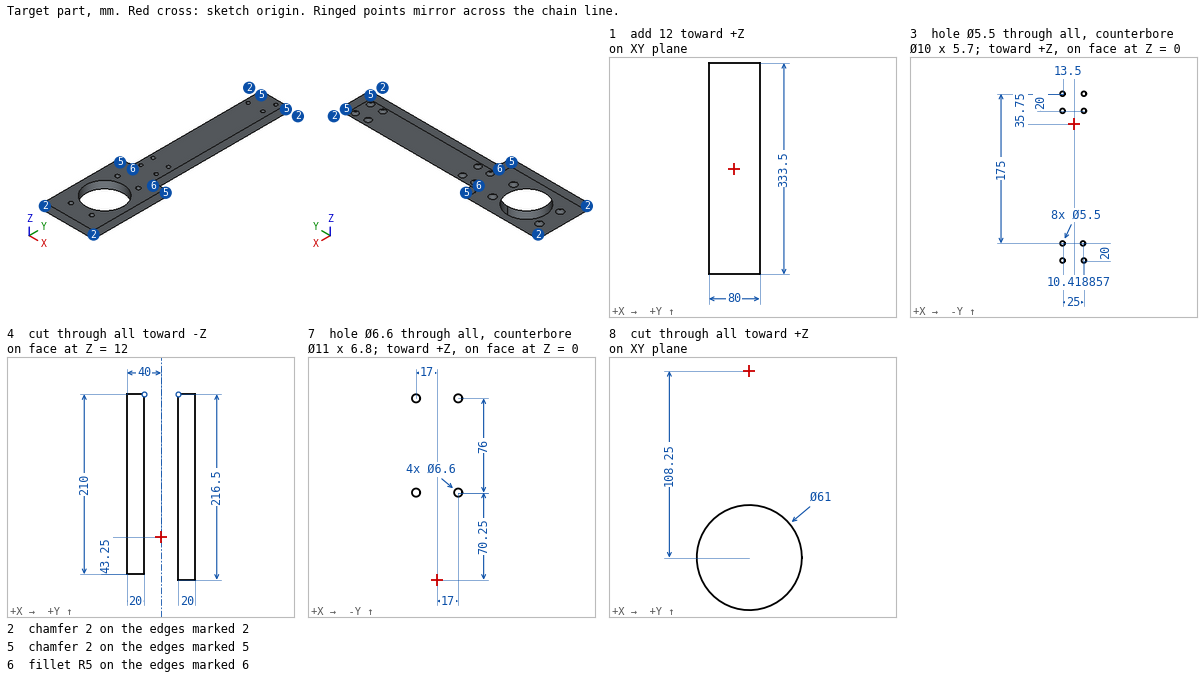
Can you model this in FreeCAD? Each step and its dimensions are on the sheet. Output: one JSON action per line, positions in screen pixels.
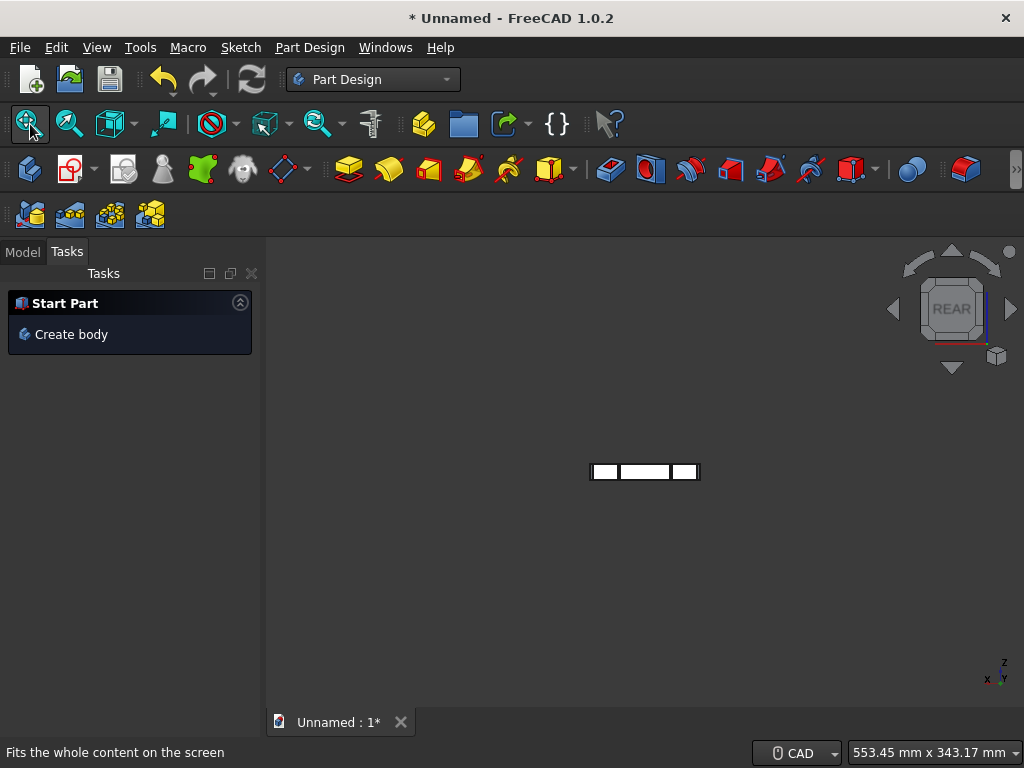
{"action": "scroll", "coordinate": [672, 471], "scroll_direction": "up", "scroll_amount": 5}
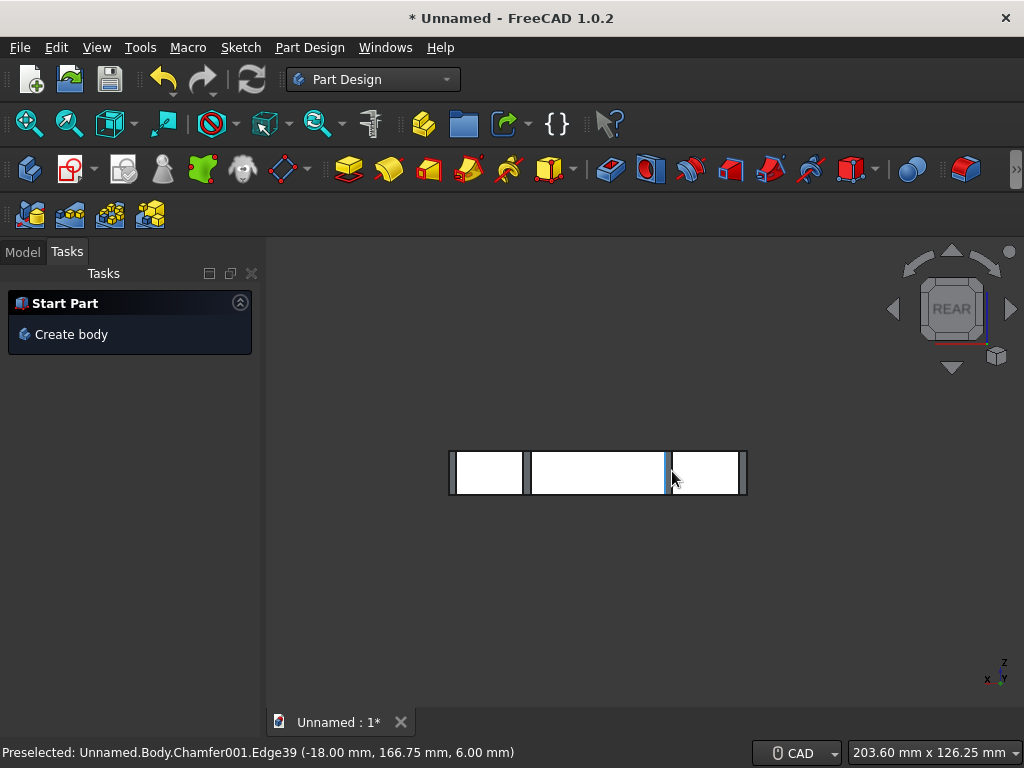
{"action": "key", "text": "v f"}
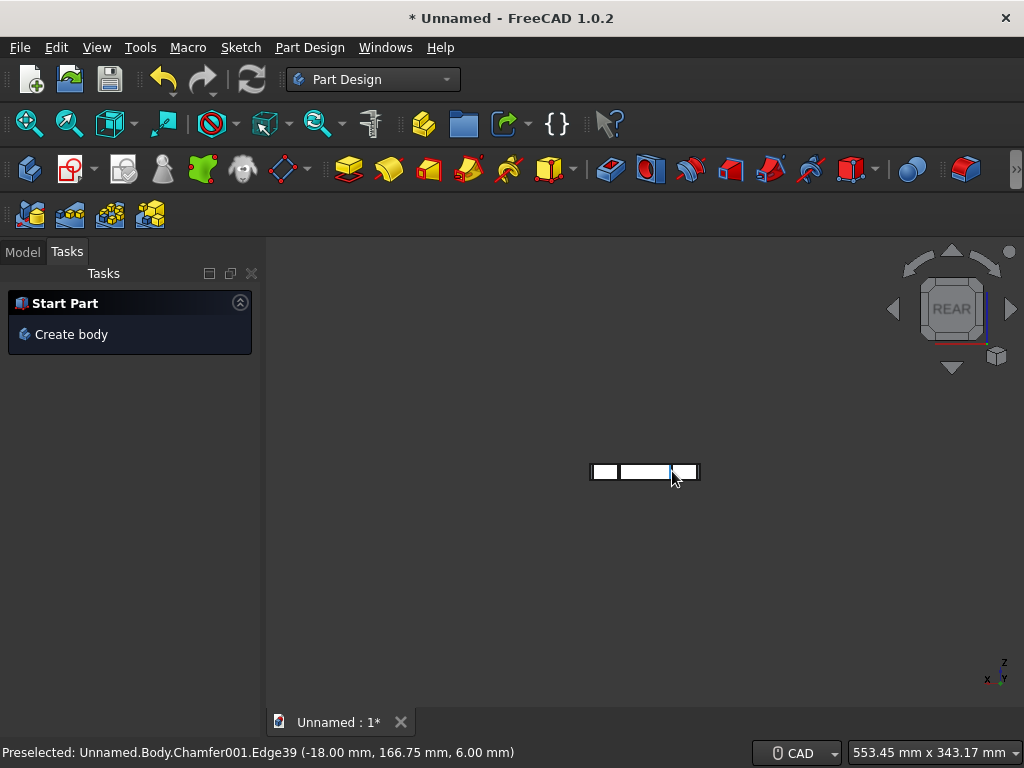
{"action": "key", "text": "6"}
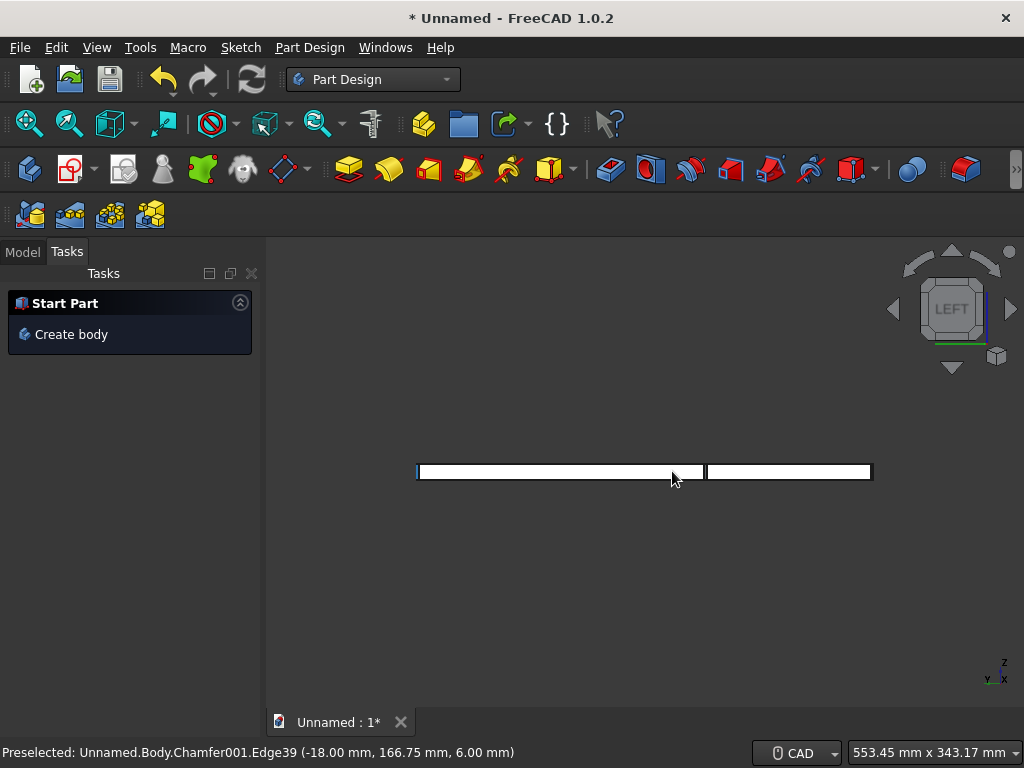
{"action": "scroll", "coordinate": [704, 471], "scroll_direction": "up", "scroll_amount": 5}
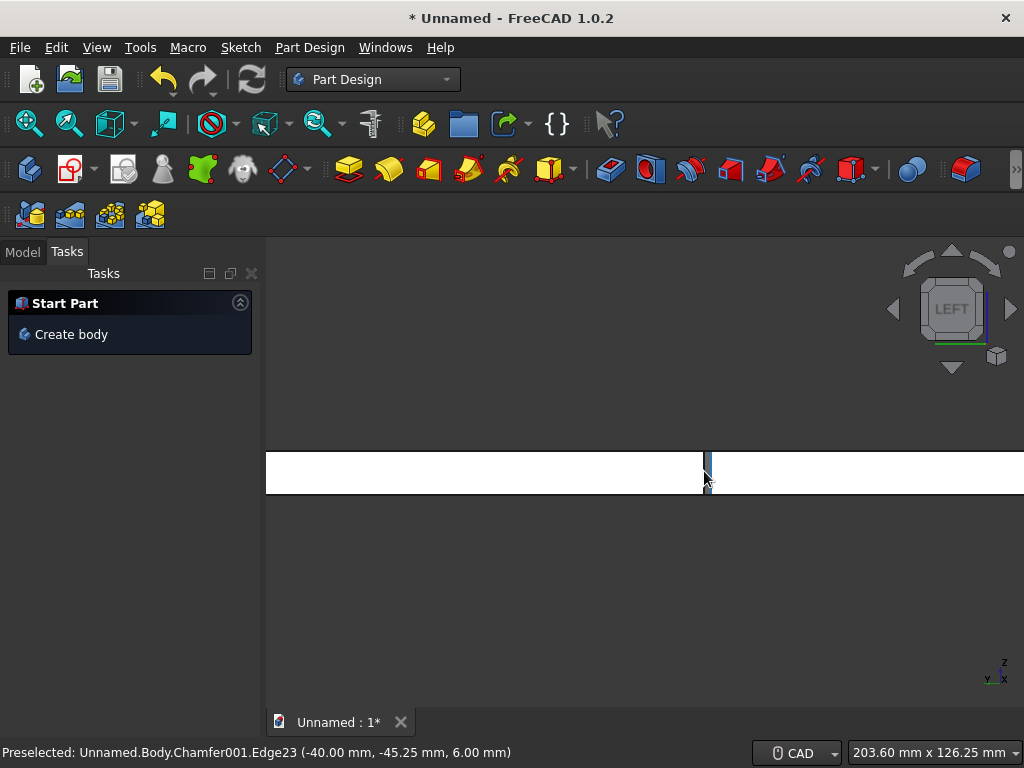
{"action": "key", "text": "v f"}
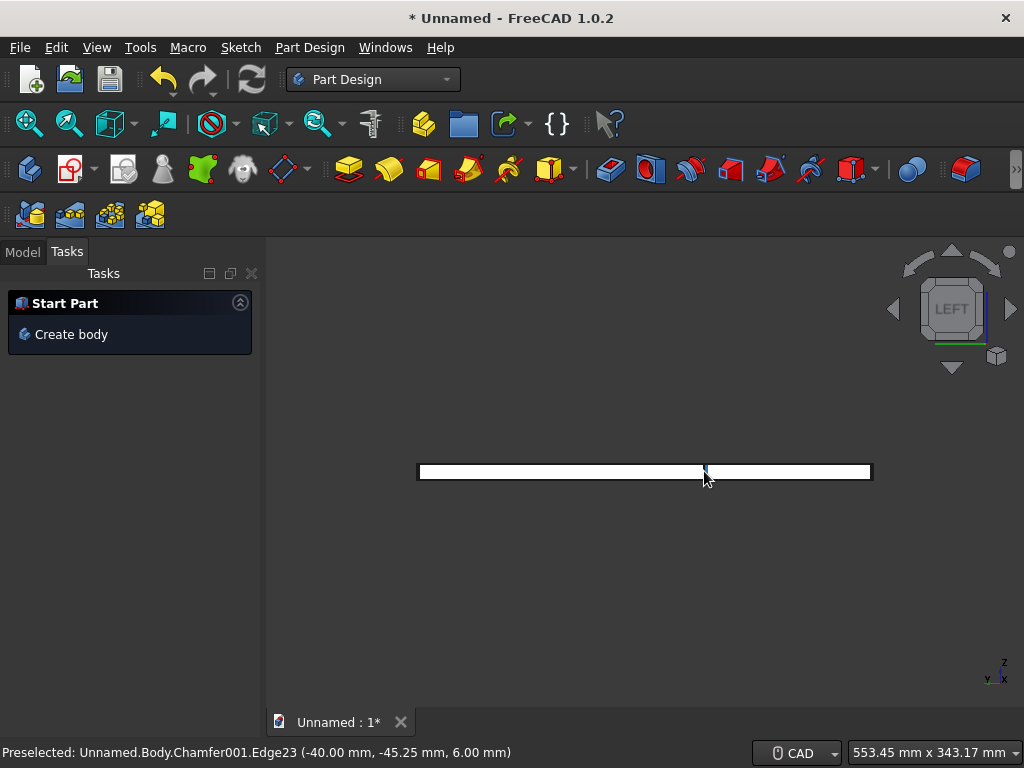
{"action": "key", "text": "v 3"}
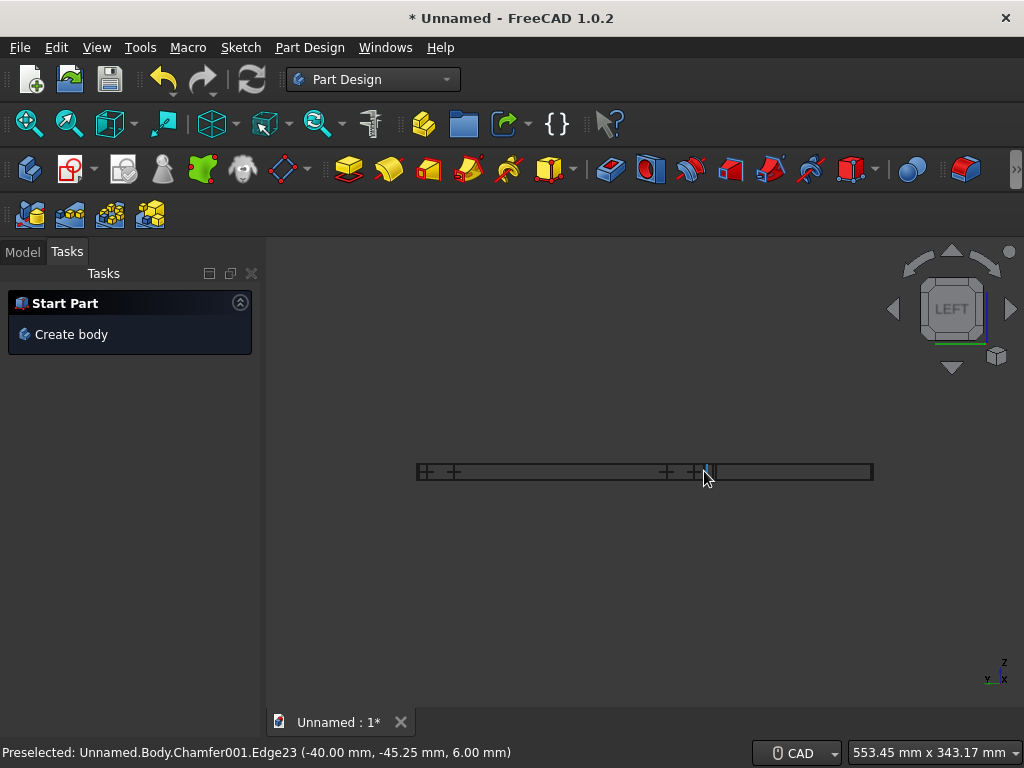
{"action": "key", "text": "0"}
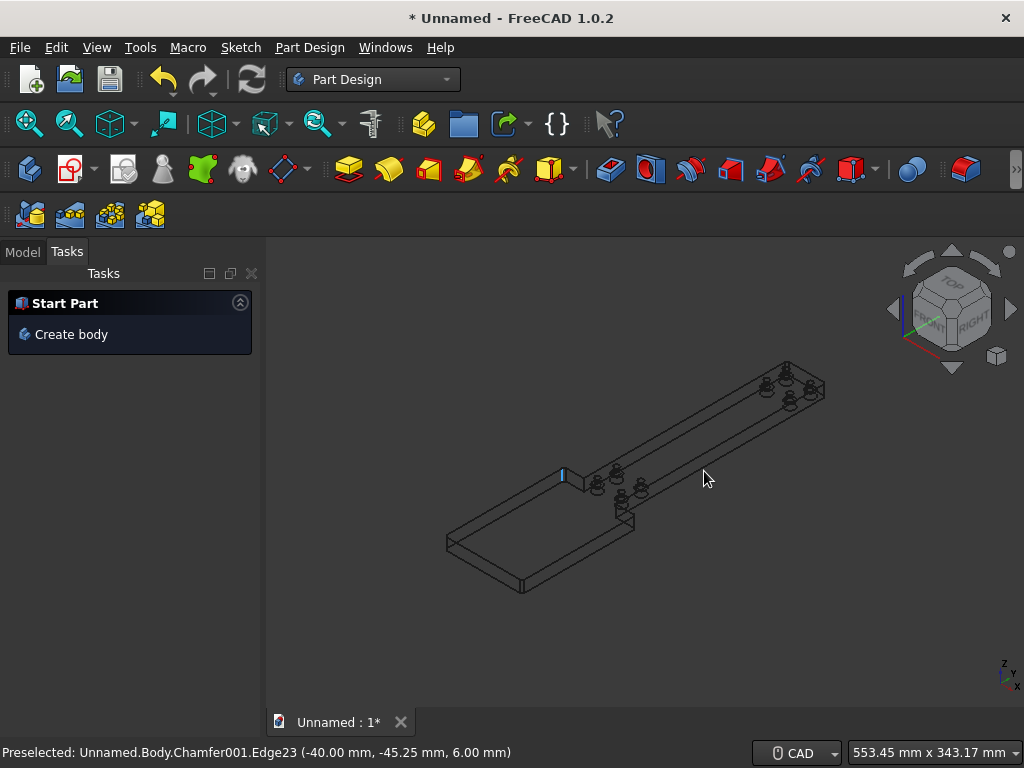
{"action": "left_click", "coordinate": [584, 484]}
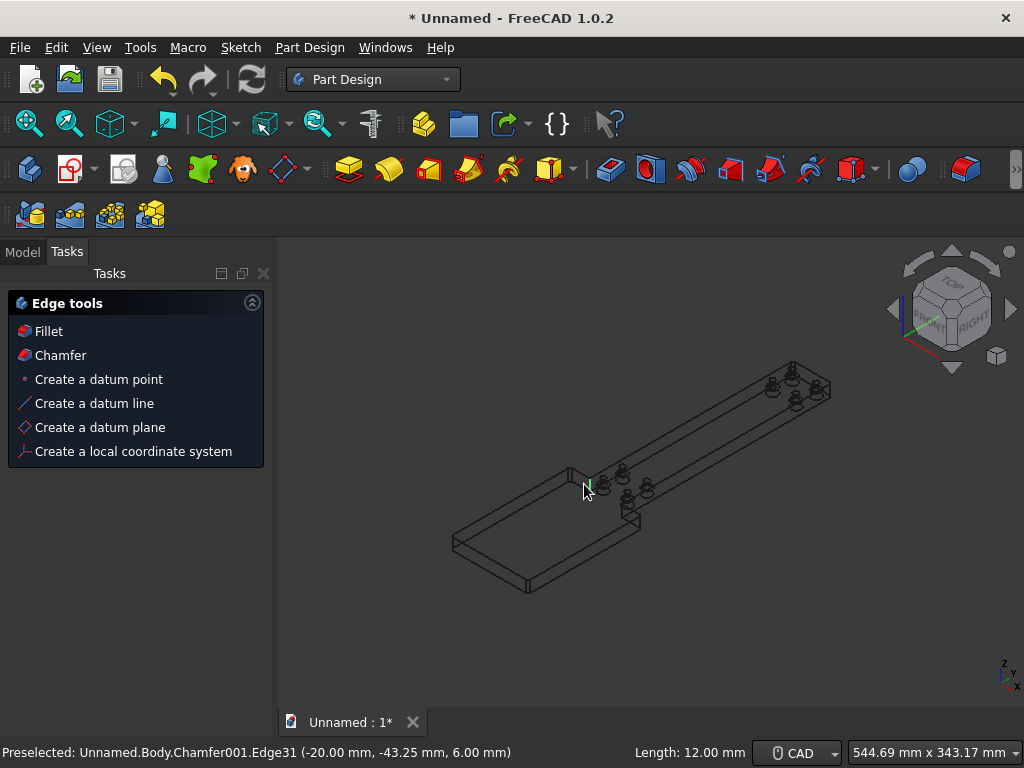
{"action": "left_click", "coordinate": [622, 511], "text": "ctrl"}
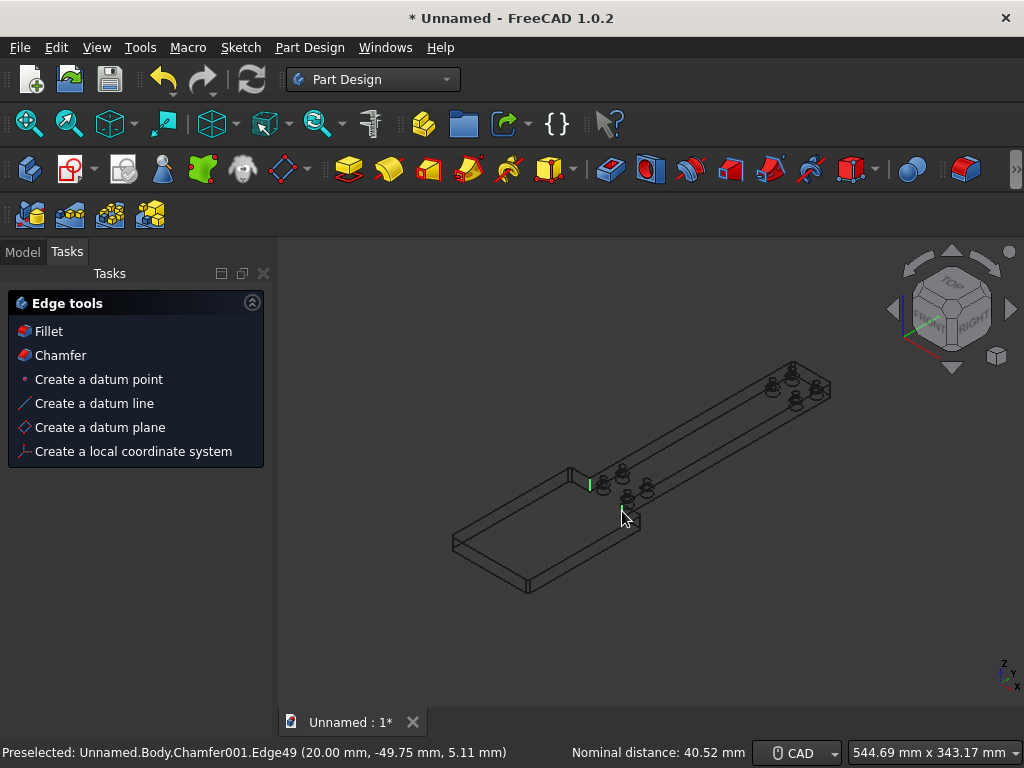
{"action": "key", "text": "v 1"}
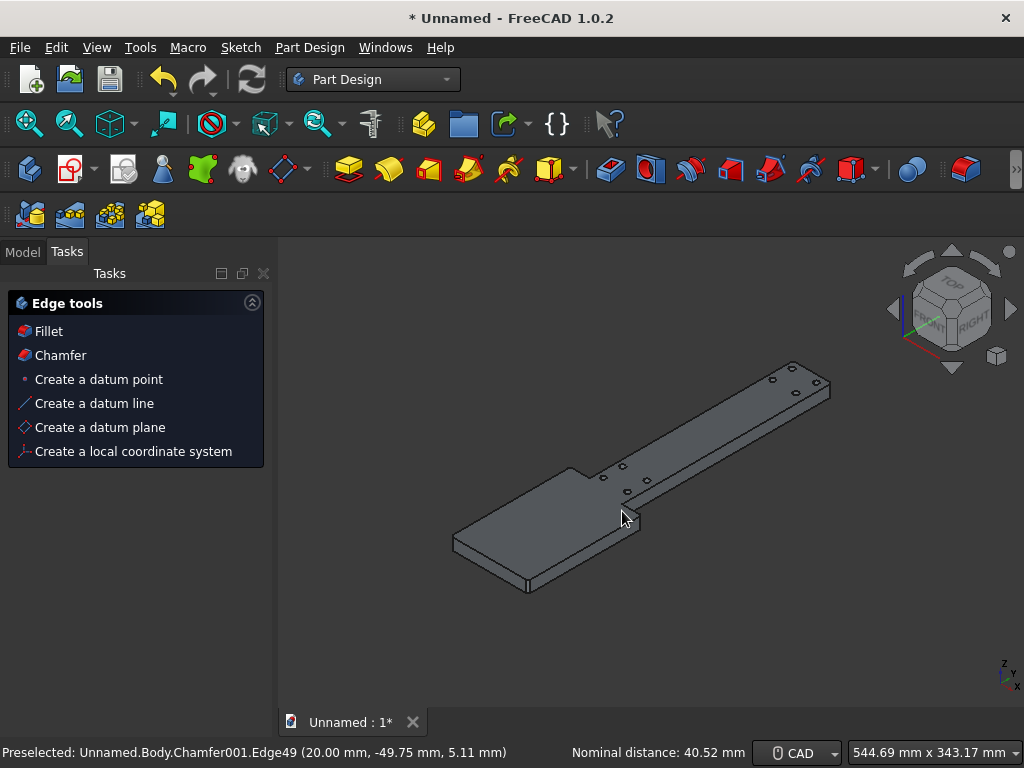
{"action": "left_click", "coordinate": [966, 170]}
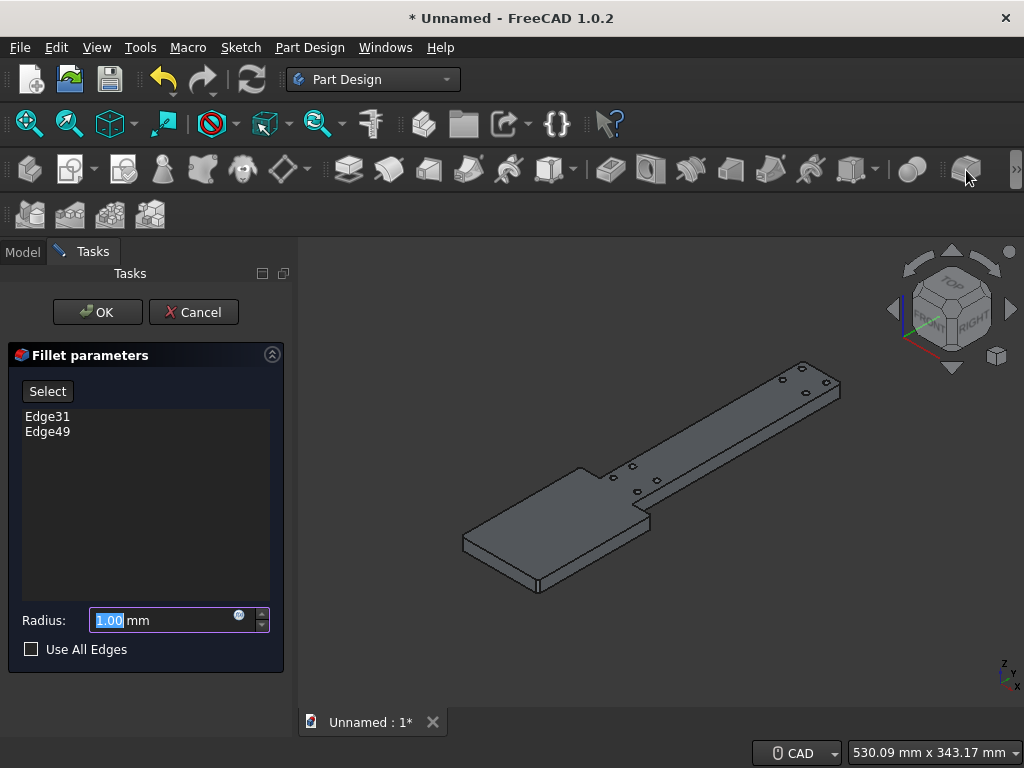
{"action": "type", "text": "5"}
{"action": "key", "text": "Tab"}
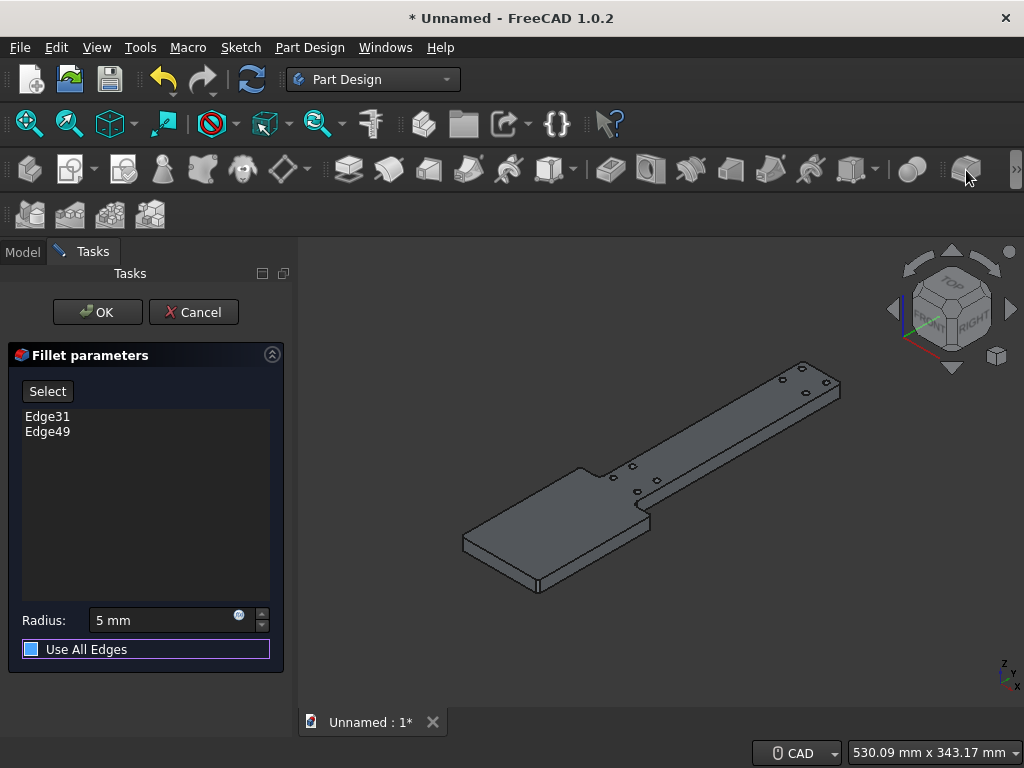
{"action": "left_click", "coordinate": [98, 312]}